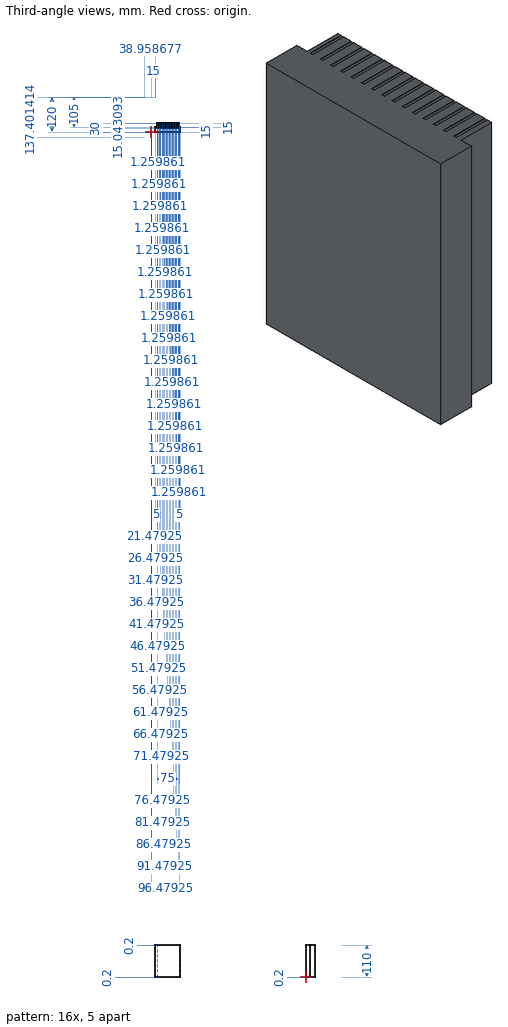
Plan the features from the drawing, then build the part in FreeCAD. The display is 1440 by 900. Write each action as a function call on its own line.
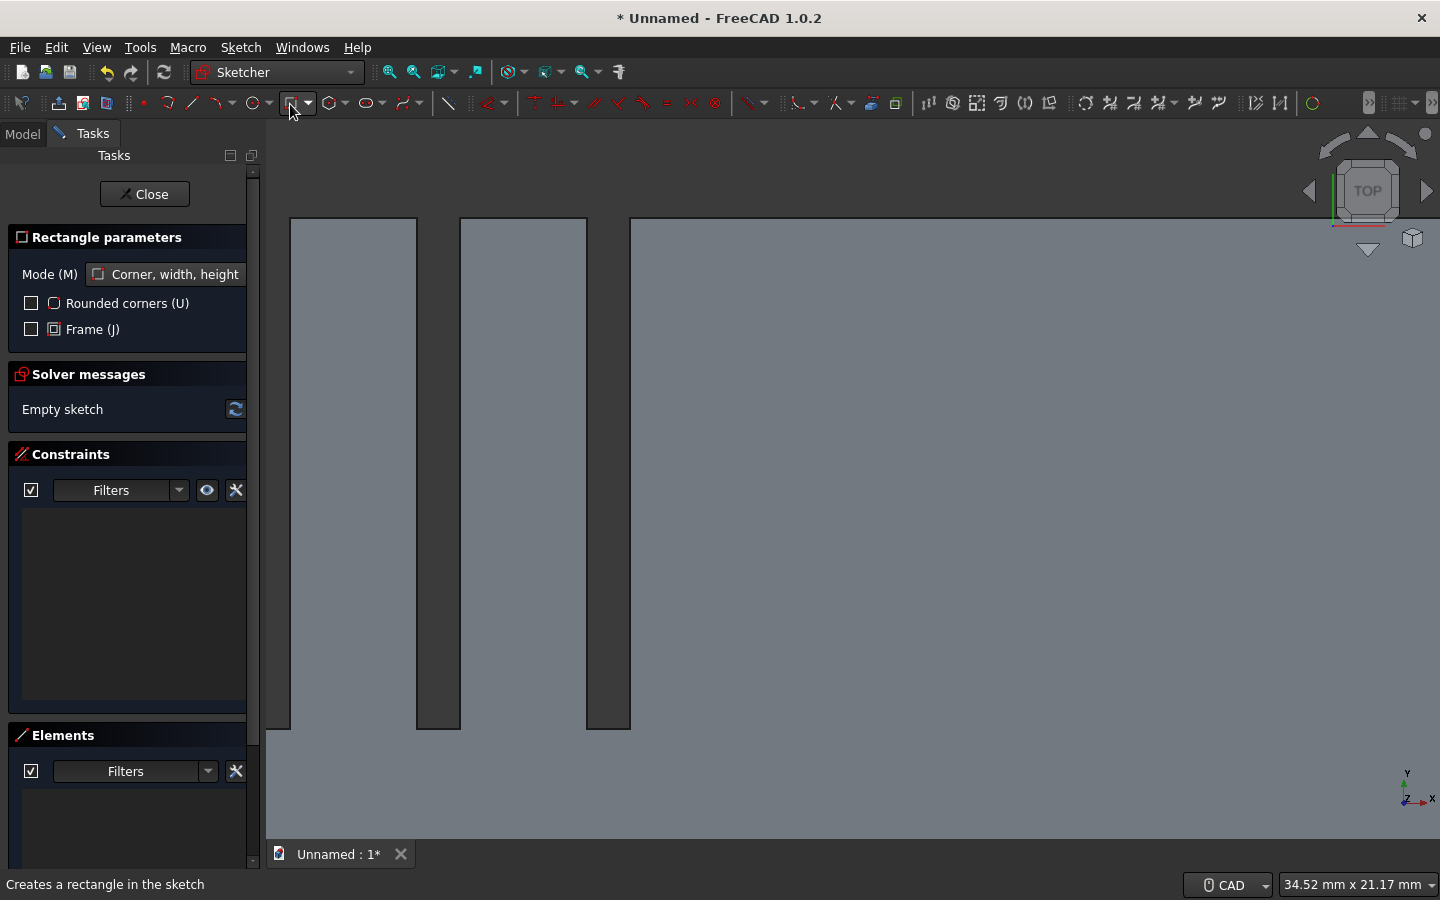
click(758, 218)
click(800, 729)
key(Escape)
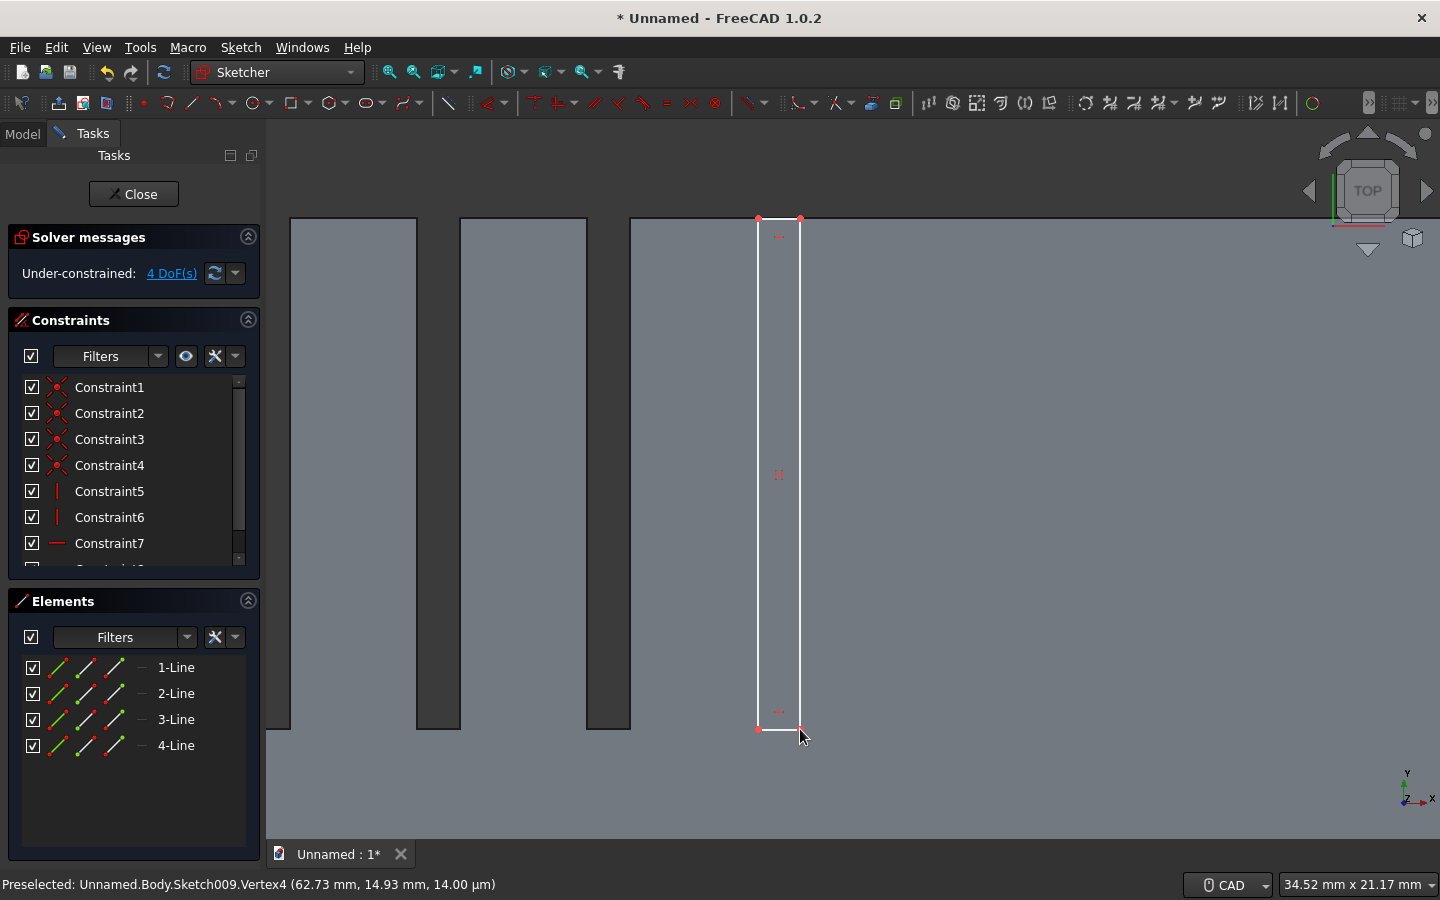
key(d)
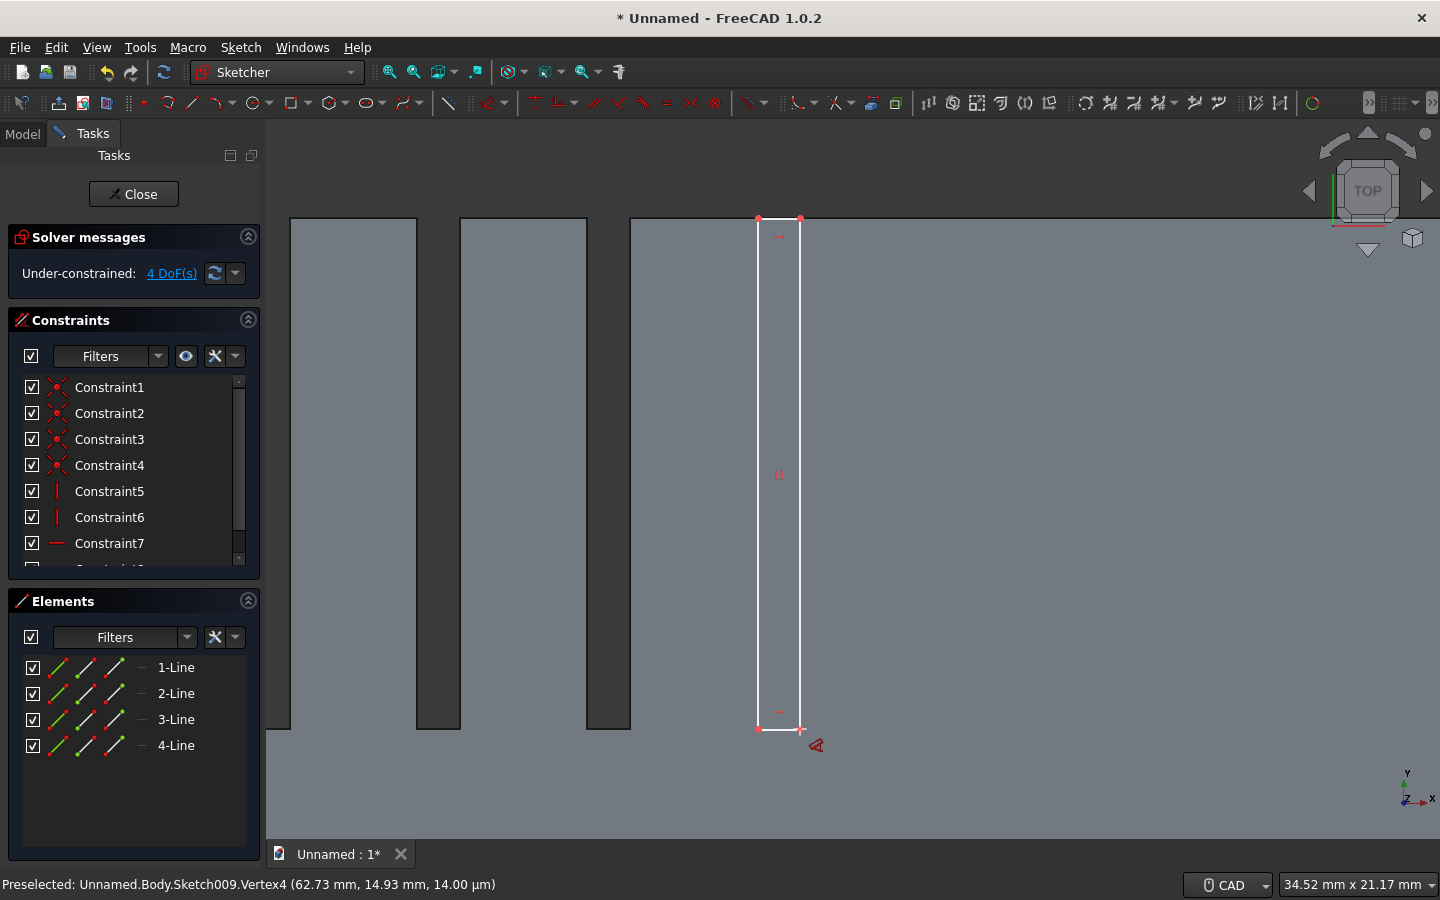
click(758, 219)
click(816, 515)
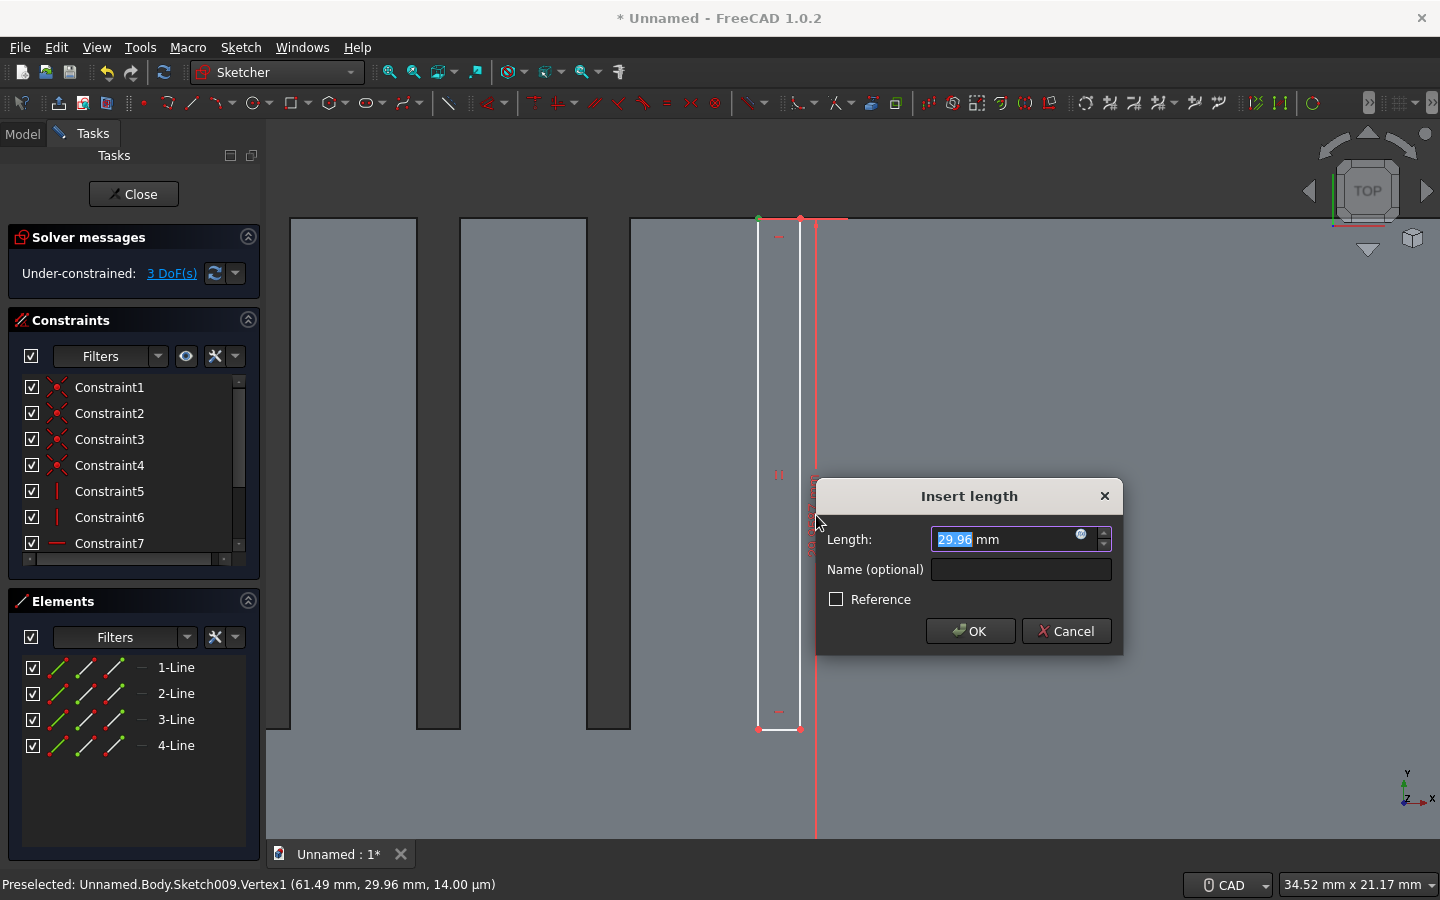
text(30)
key(Return)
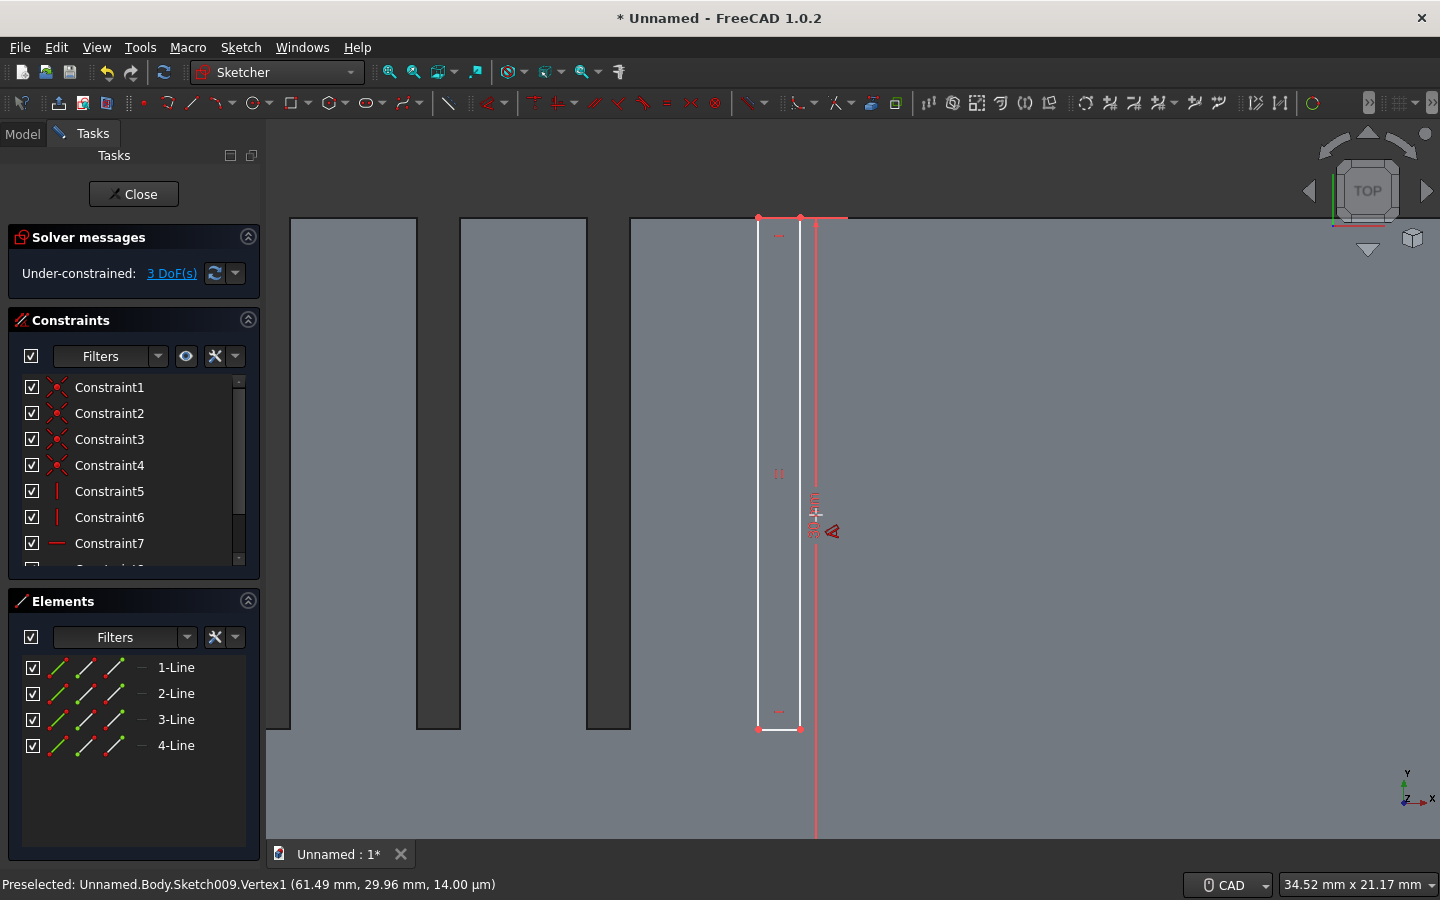
click(771, 730)
click(779, 764)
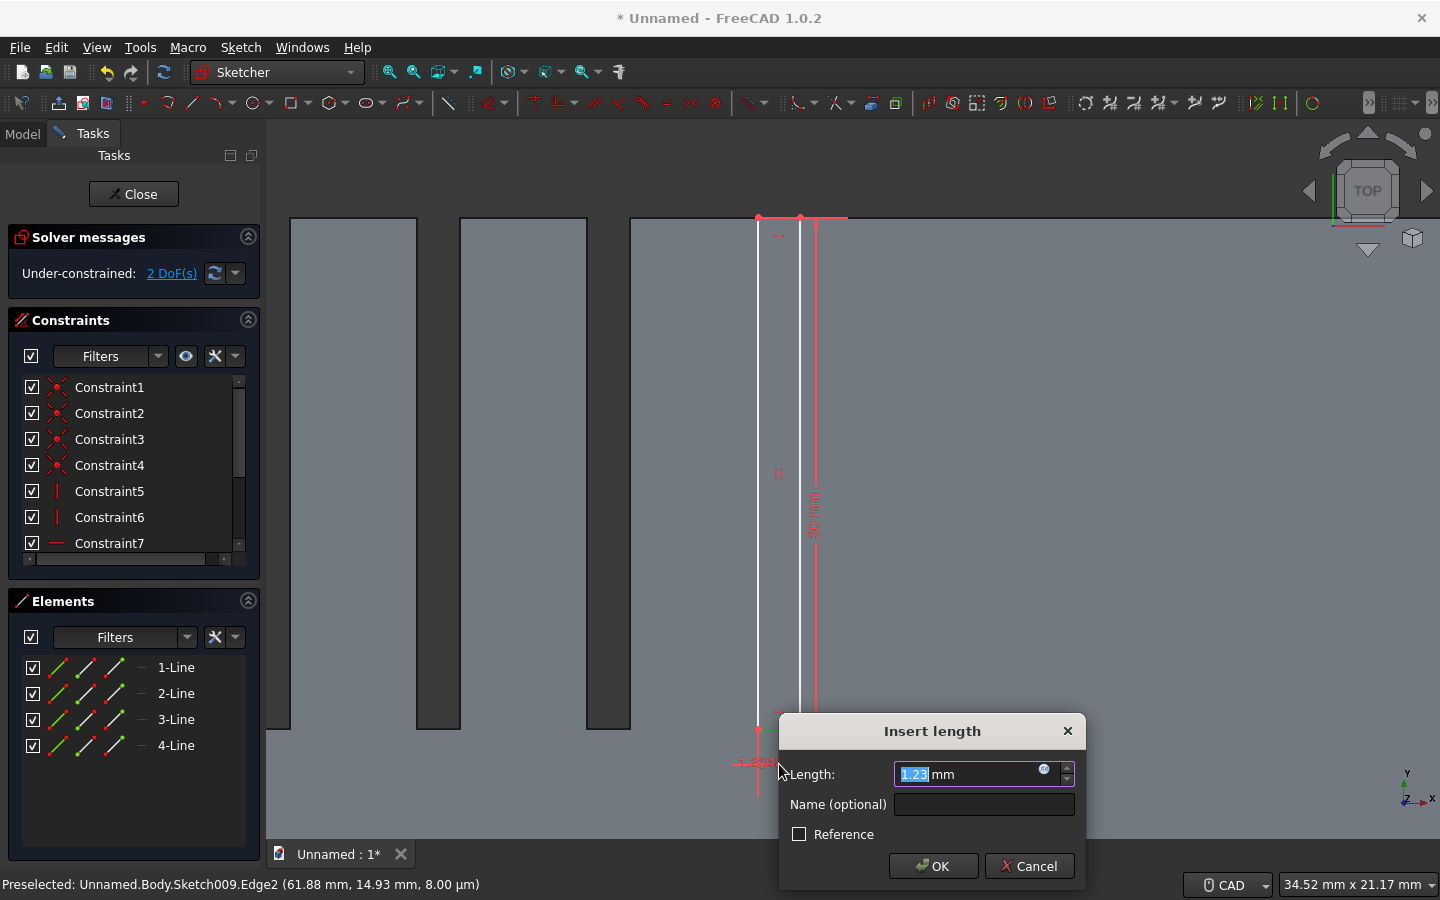
text(1.259861)
key(Return)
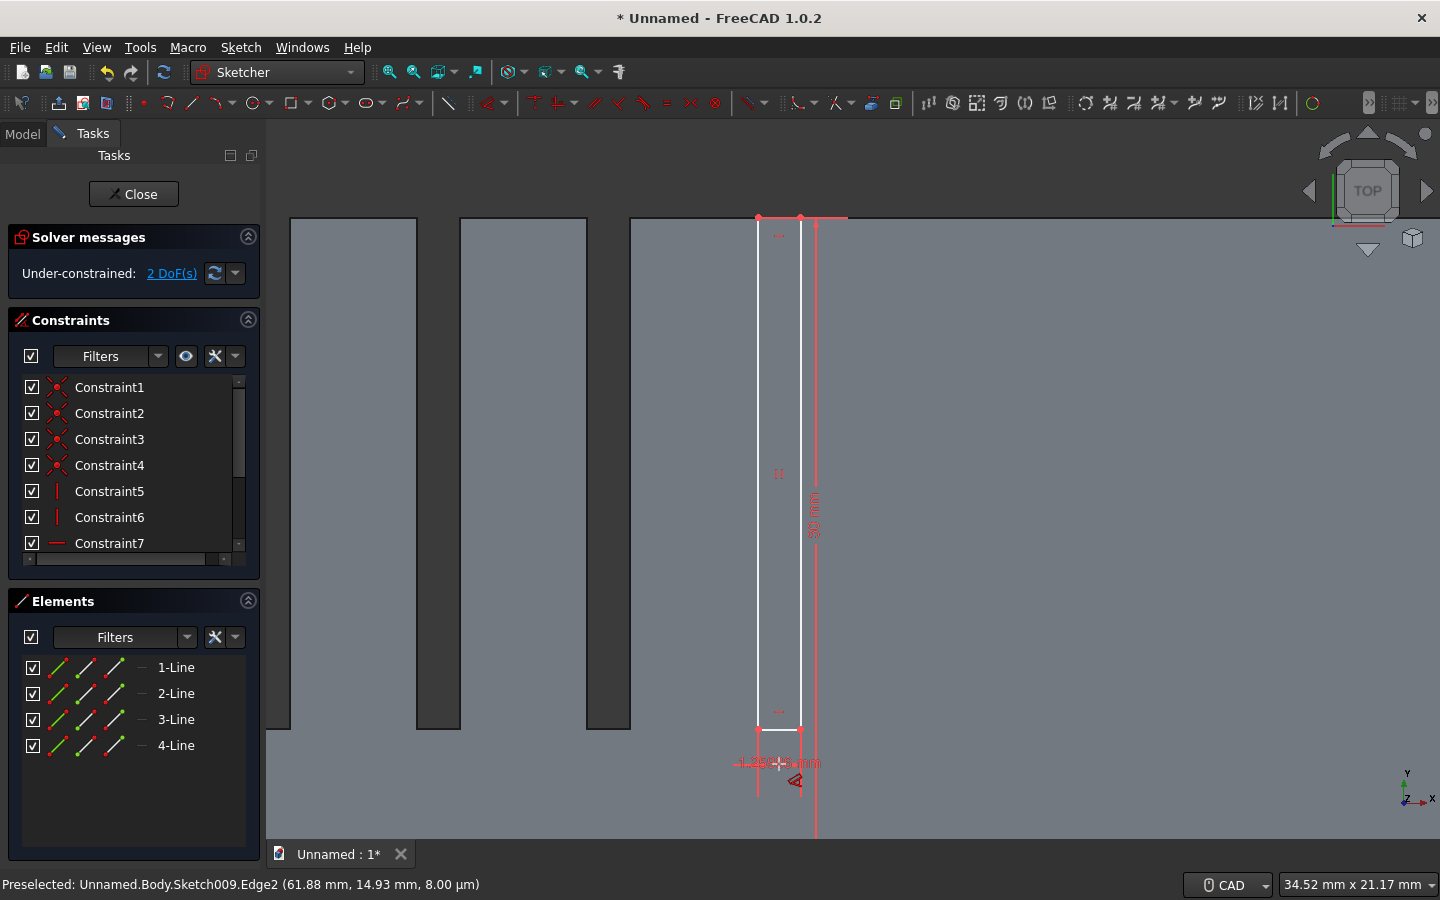
click(758, 371)
click(724, 474)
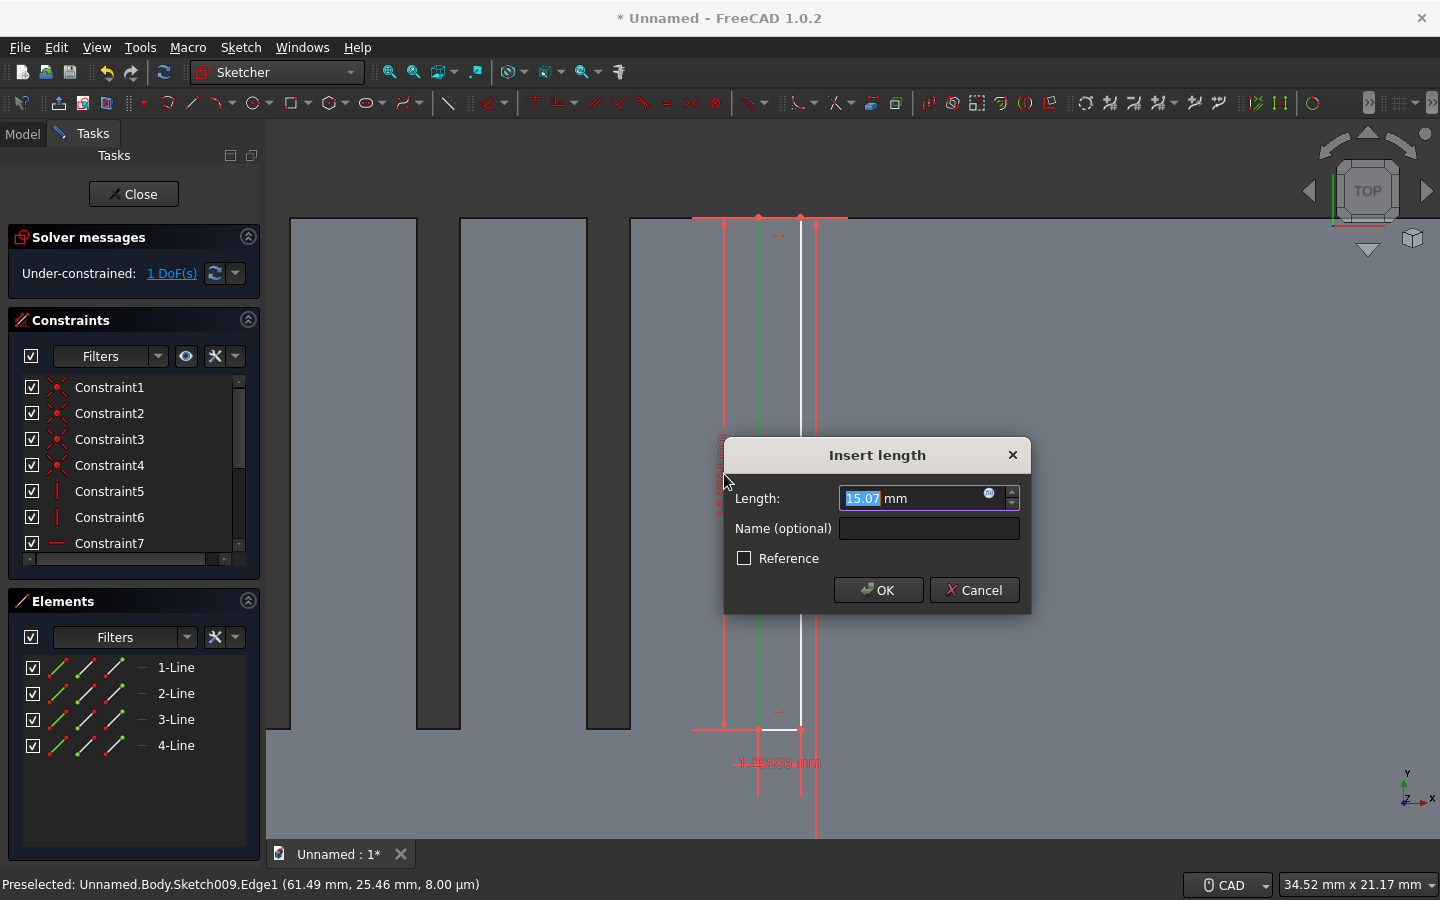
text(15.043093)
key(Return)